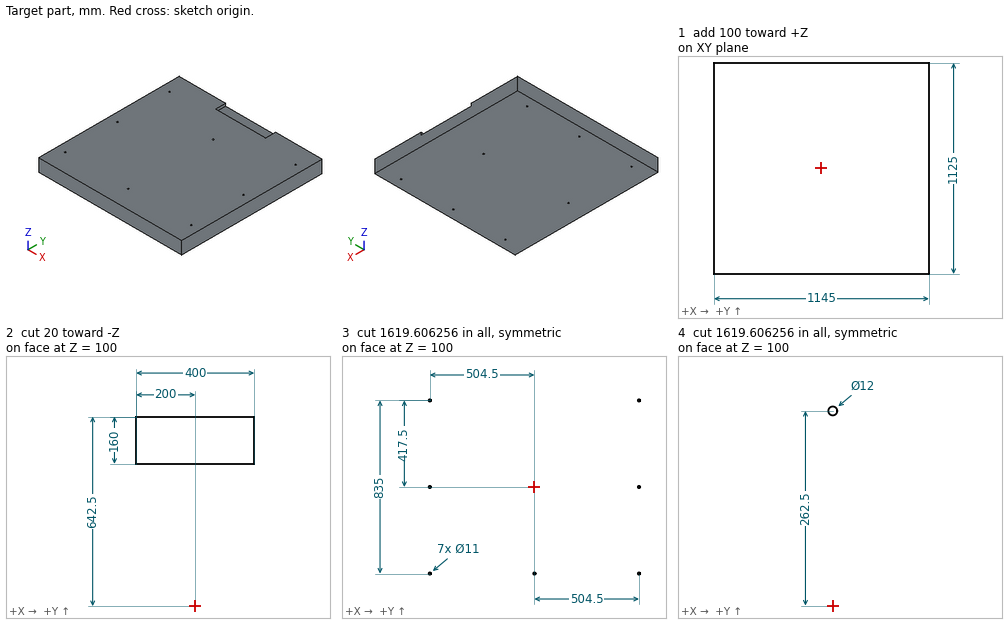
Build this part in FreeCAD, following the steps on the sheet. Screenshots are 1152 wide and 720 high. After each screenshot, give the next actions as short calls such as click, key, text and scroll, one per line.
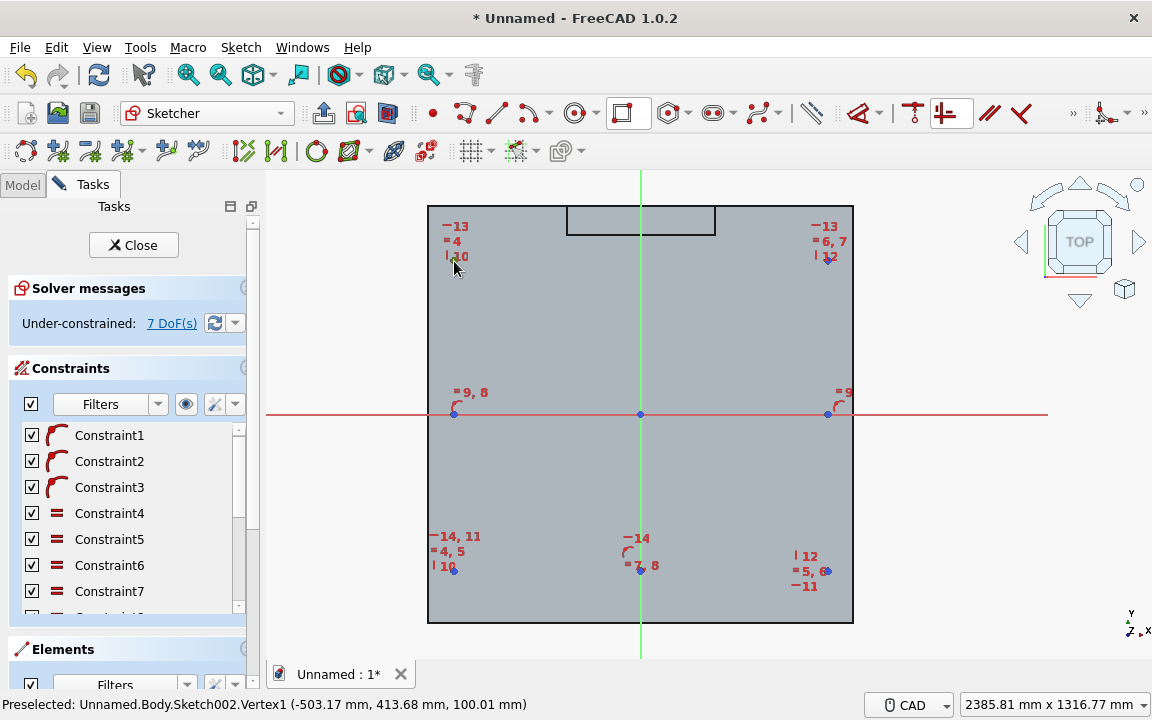
click(454, 415)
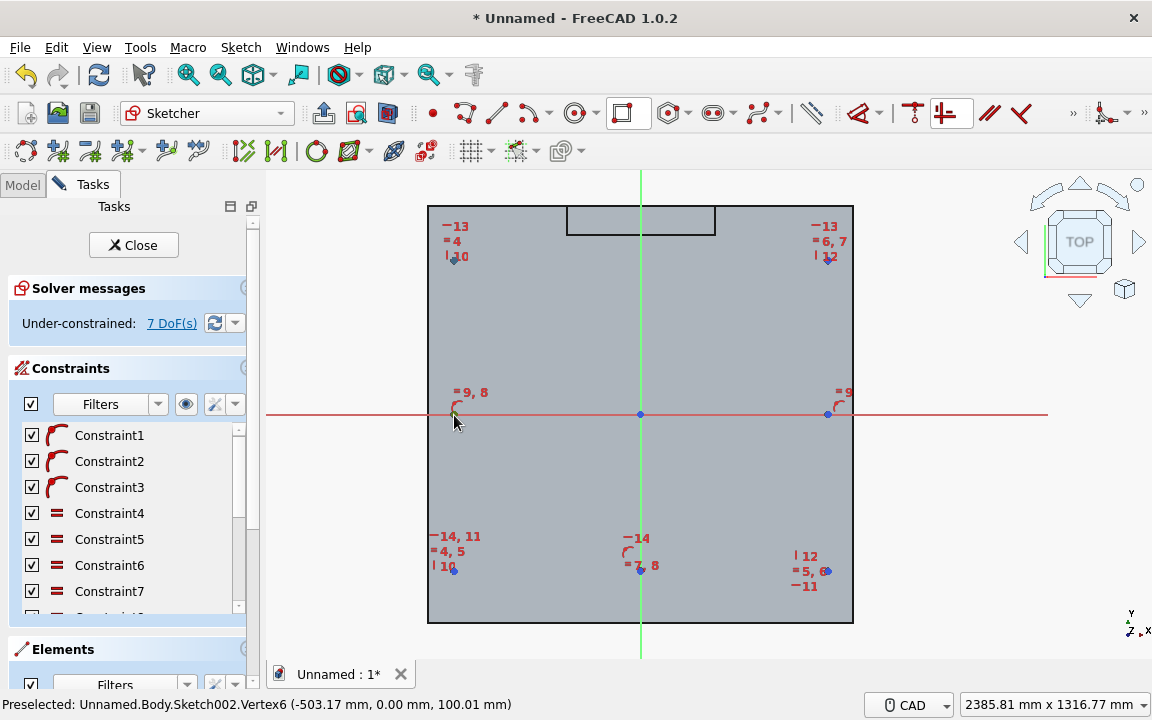
key(v)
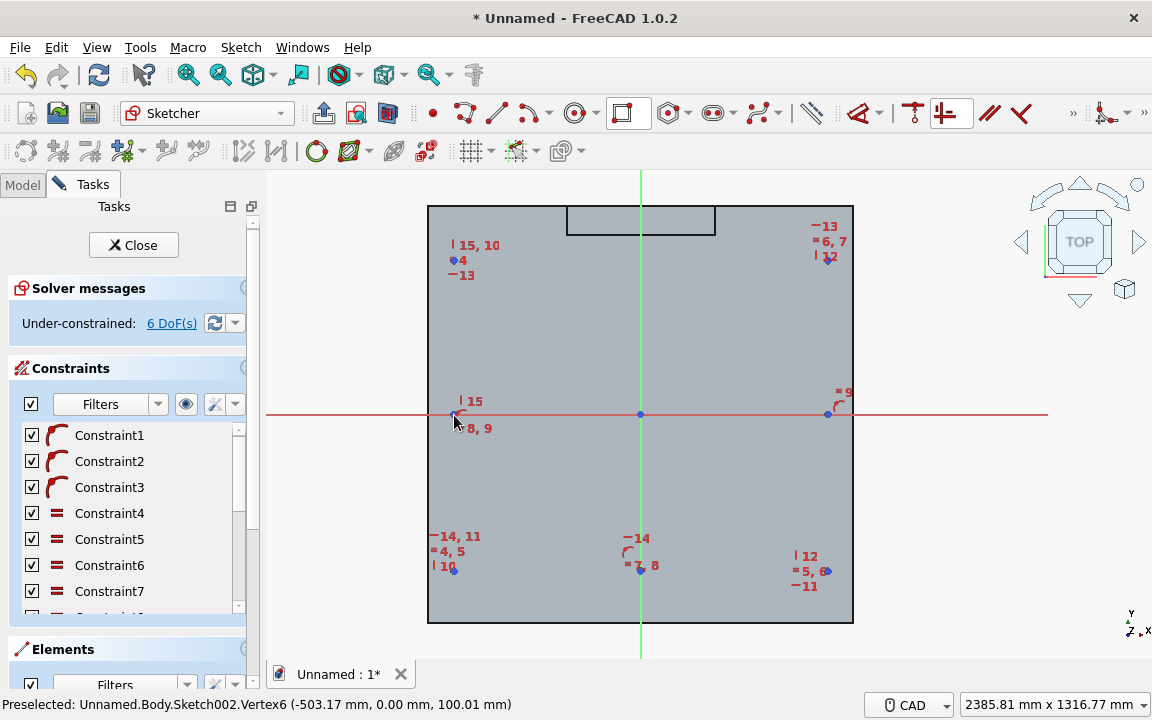
click(828, 571)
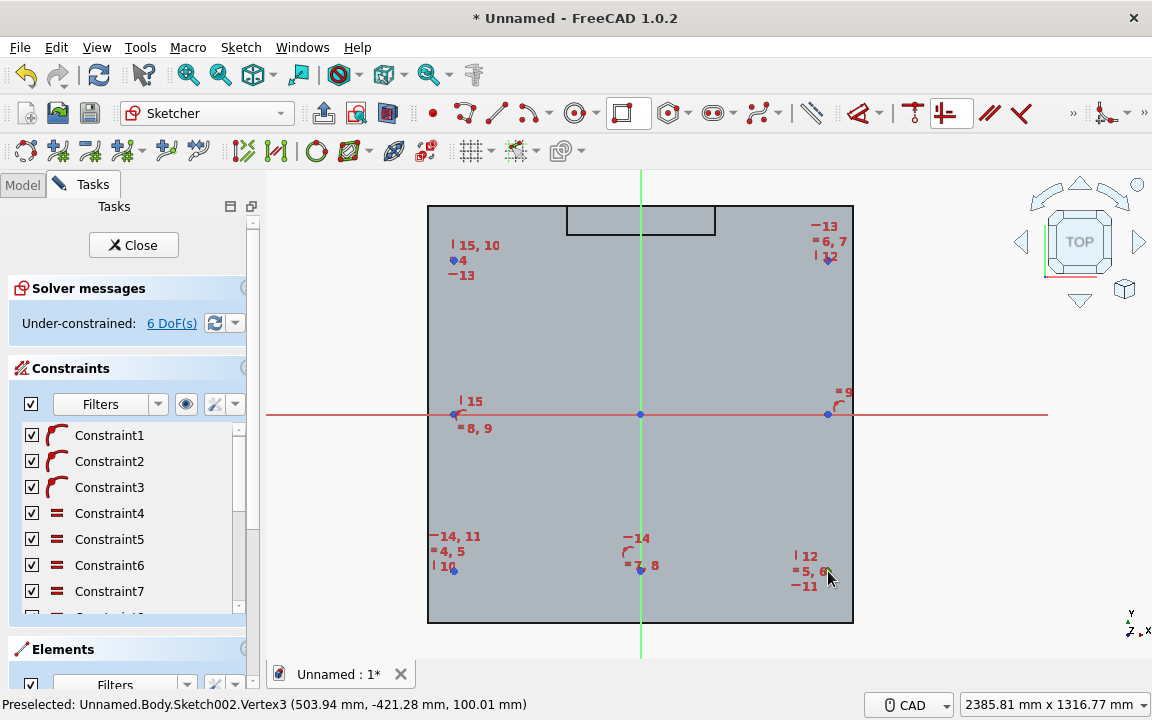
click(828, 415)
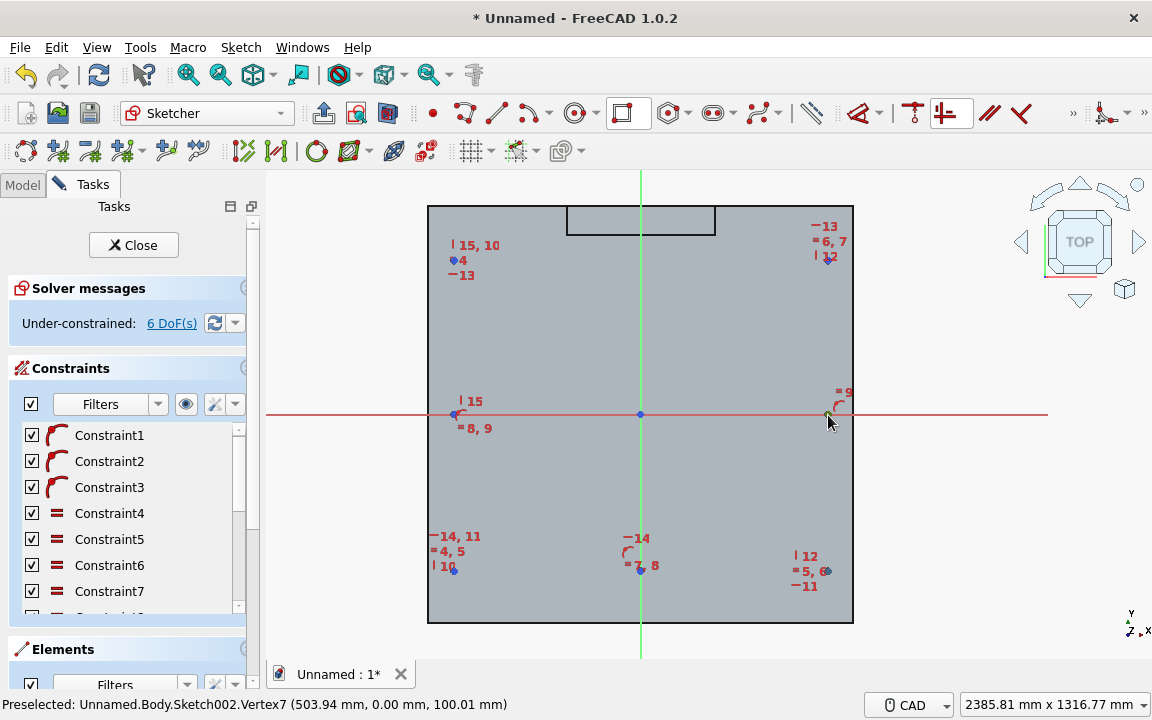
click(968, 114)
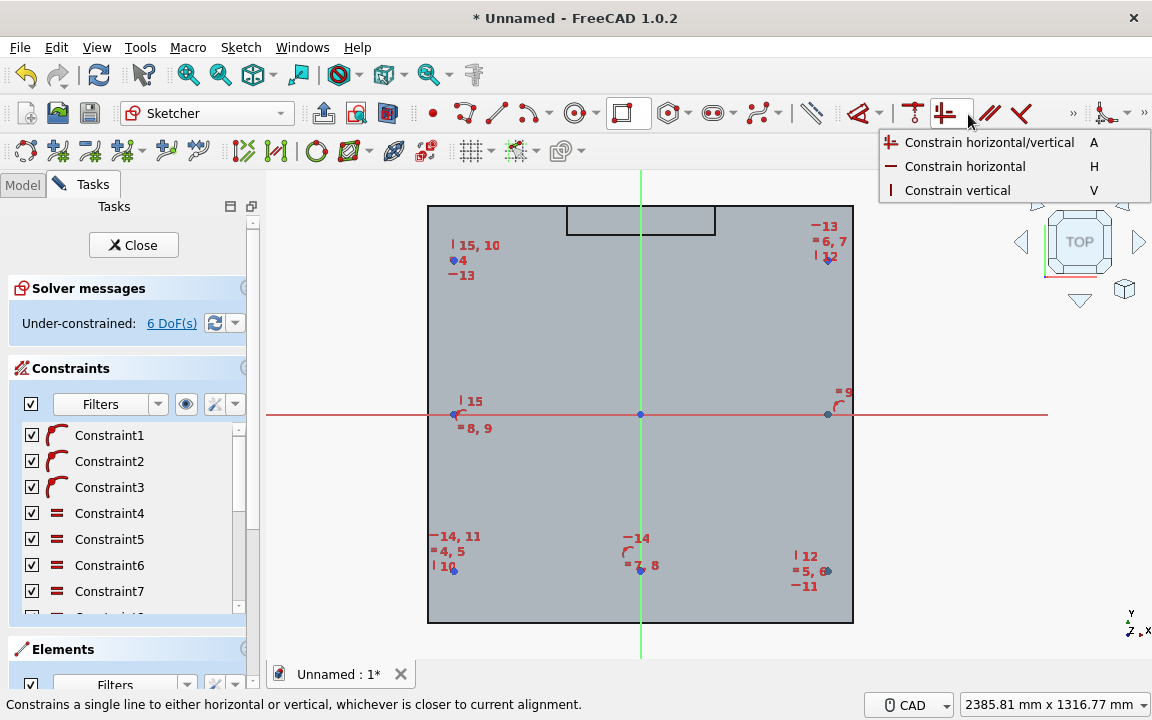
click(1015, 190)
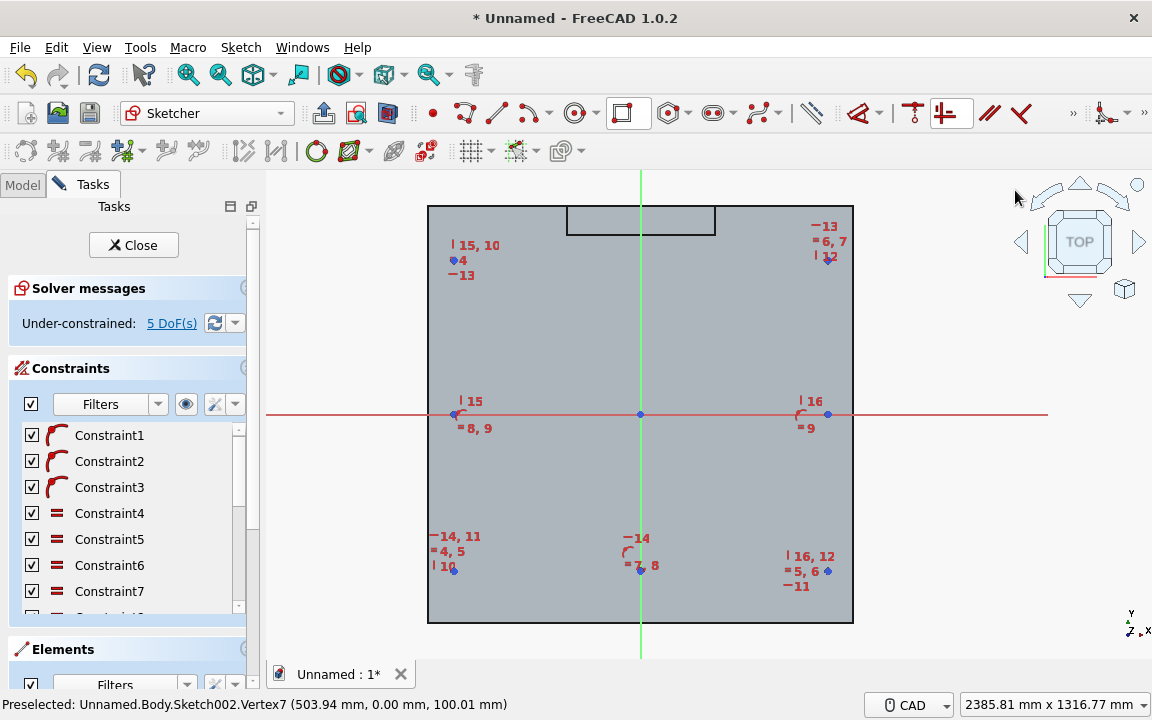
key(d)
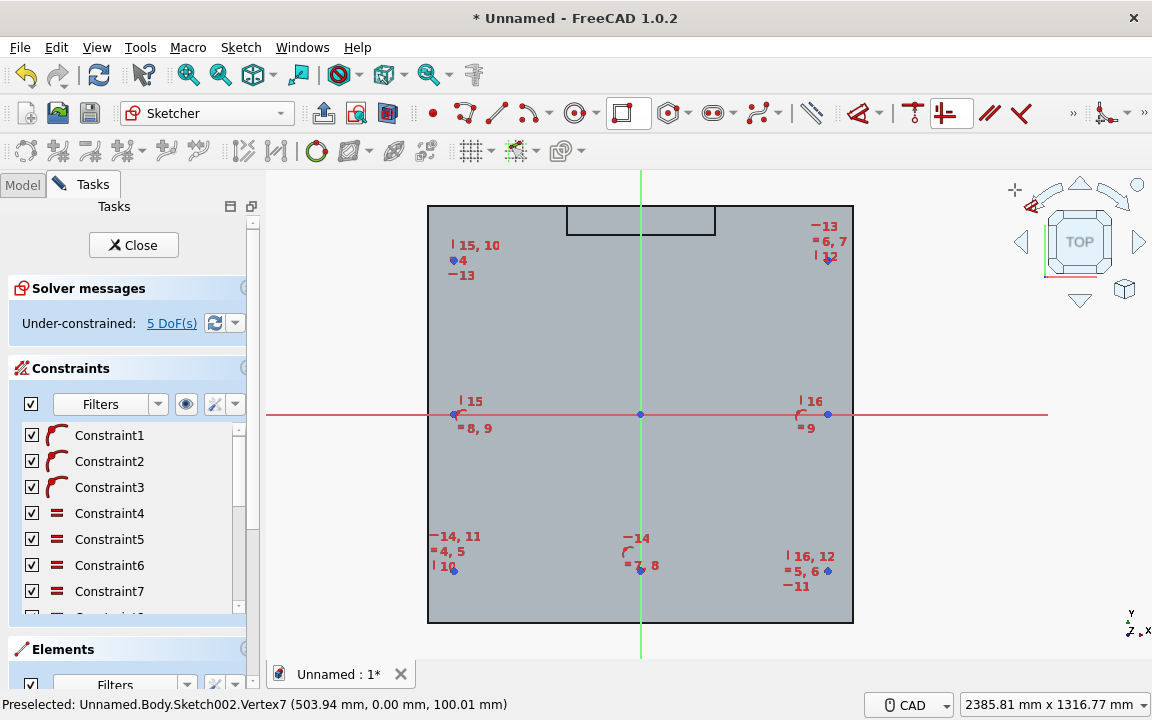
scroll(454, 258, up, 12)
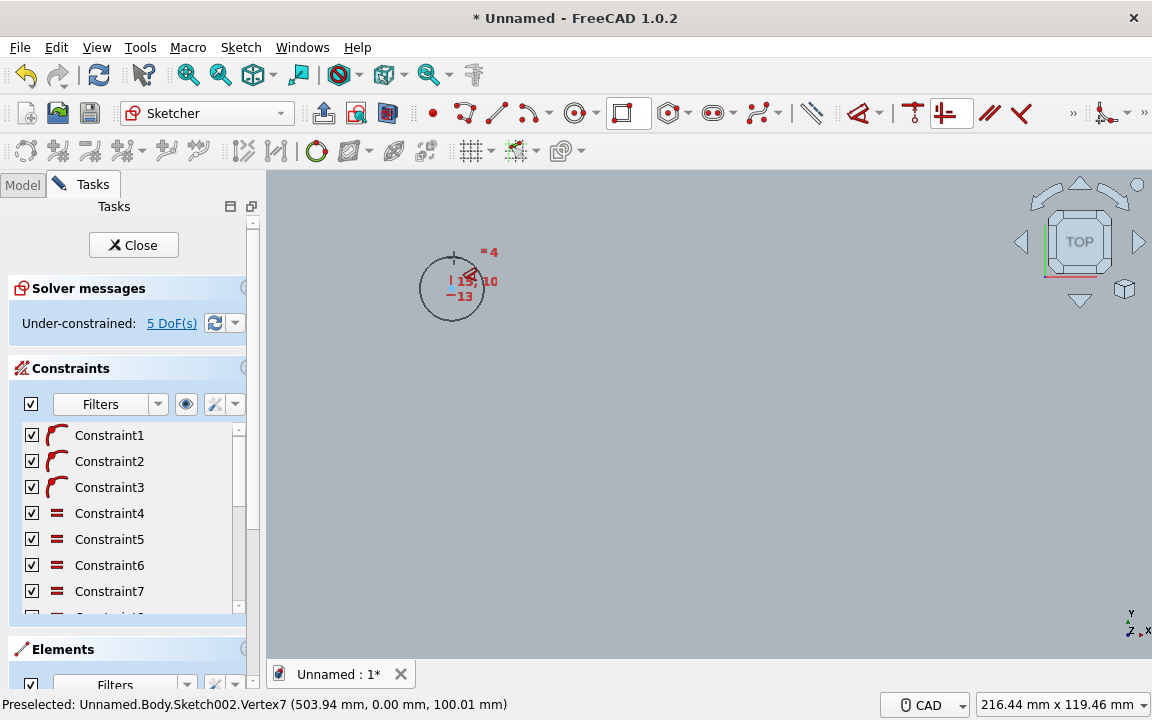
click(453, 257)
click(454, 225)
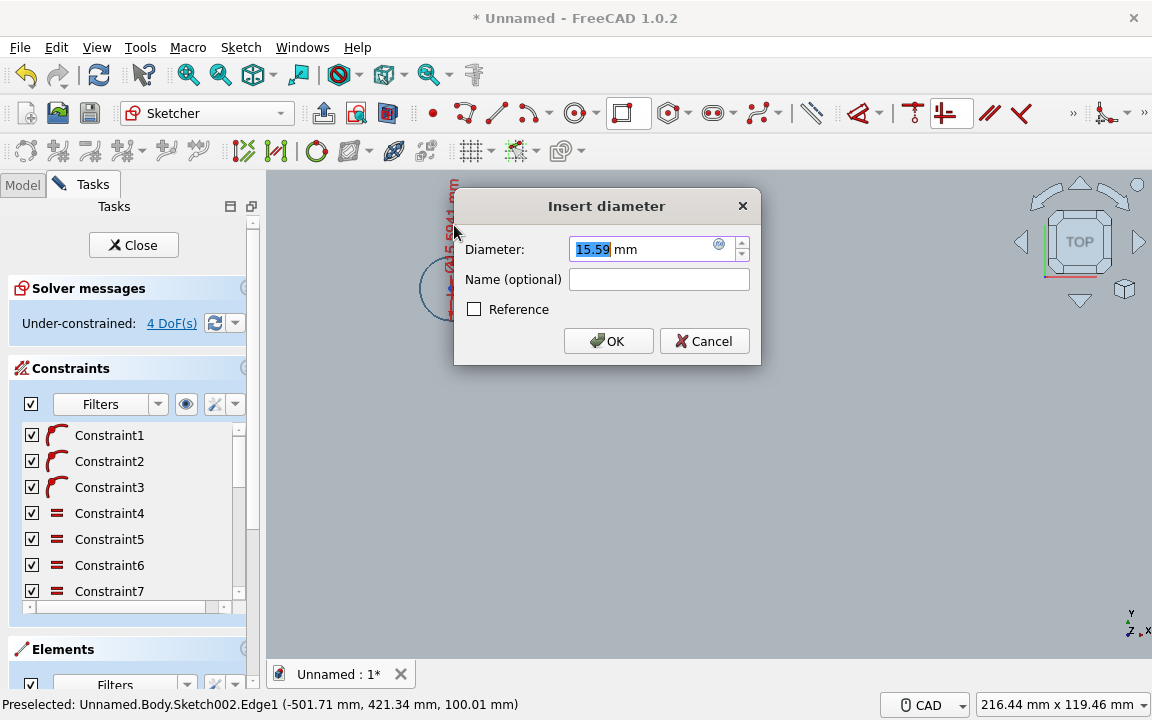
text(11)
key(Return)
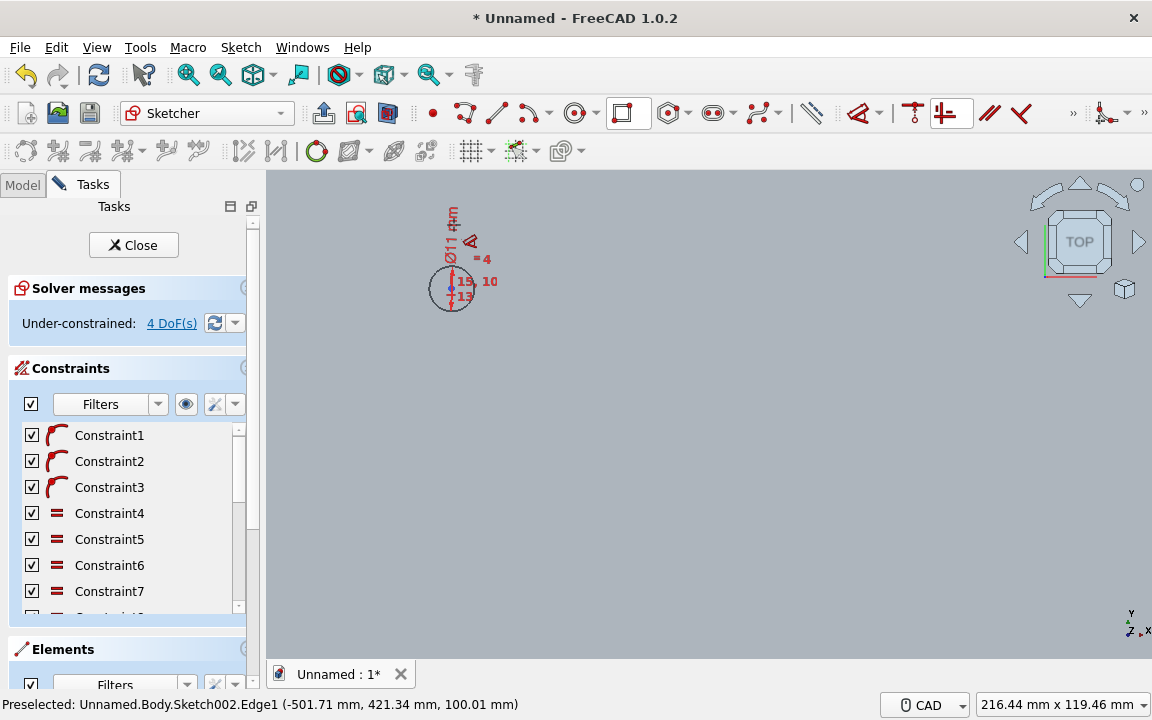
scroll(454, 258, down, 12)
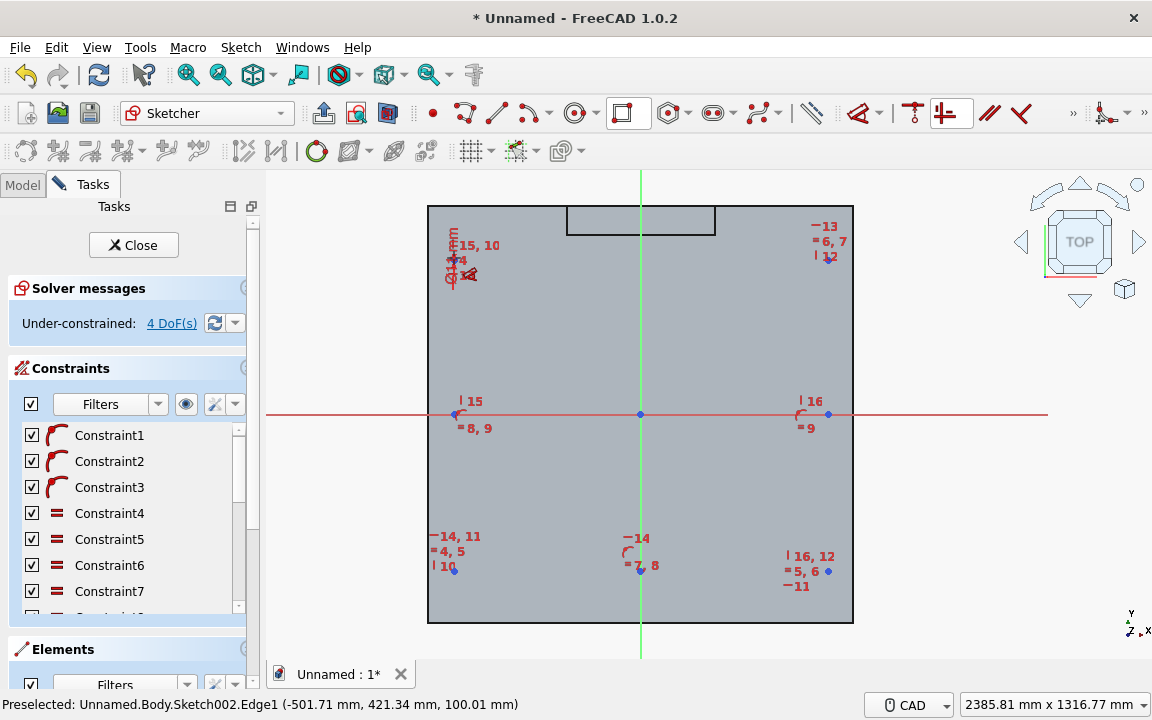
click(454, 261)